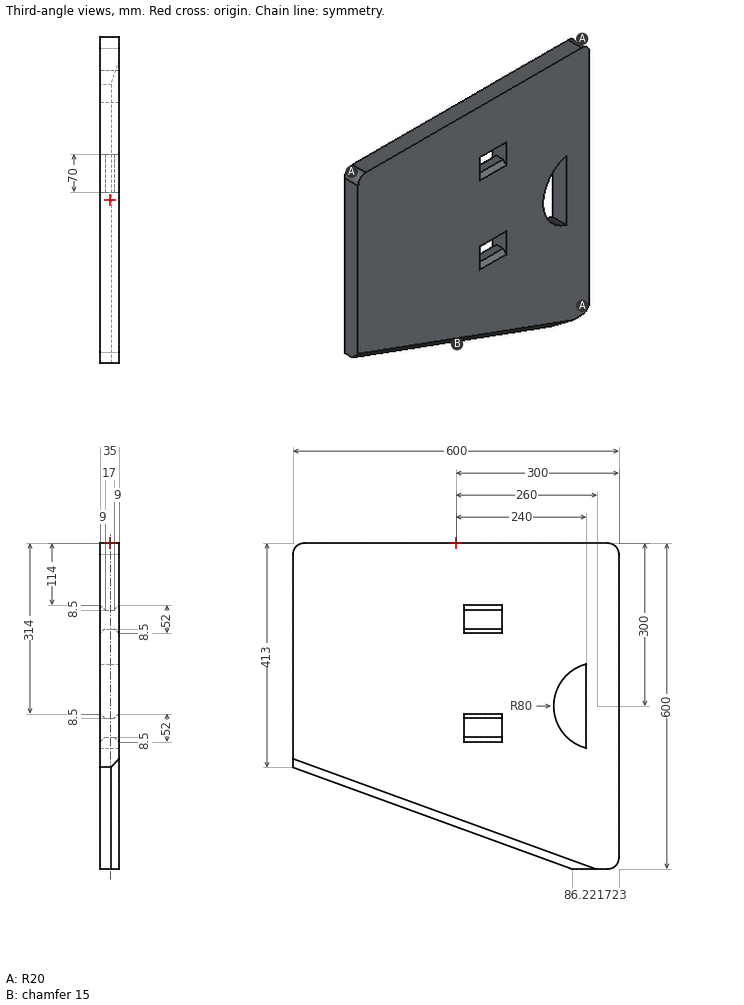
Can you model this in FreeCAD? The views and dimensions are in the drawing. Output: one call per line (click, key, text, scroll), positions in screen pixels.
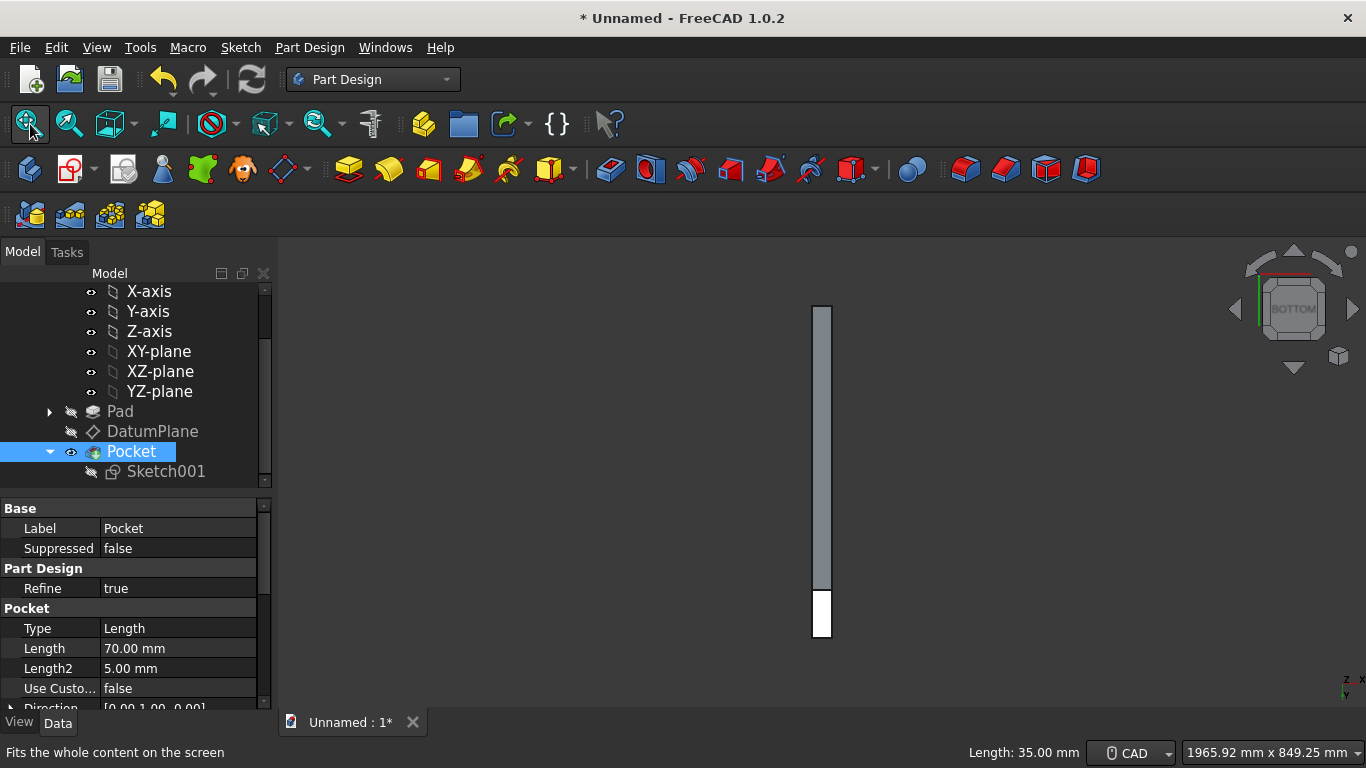
click(822, 637, ctrl)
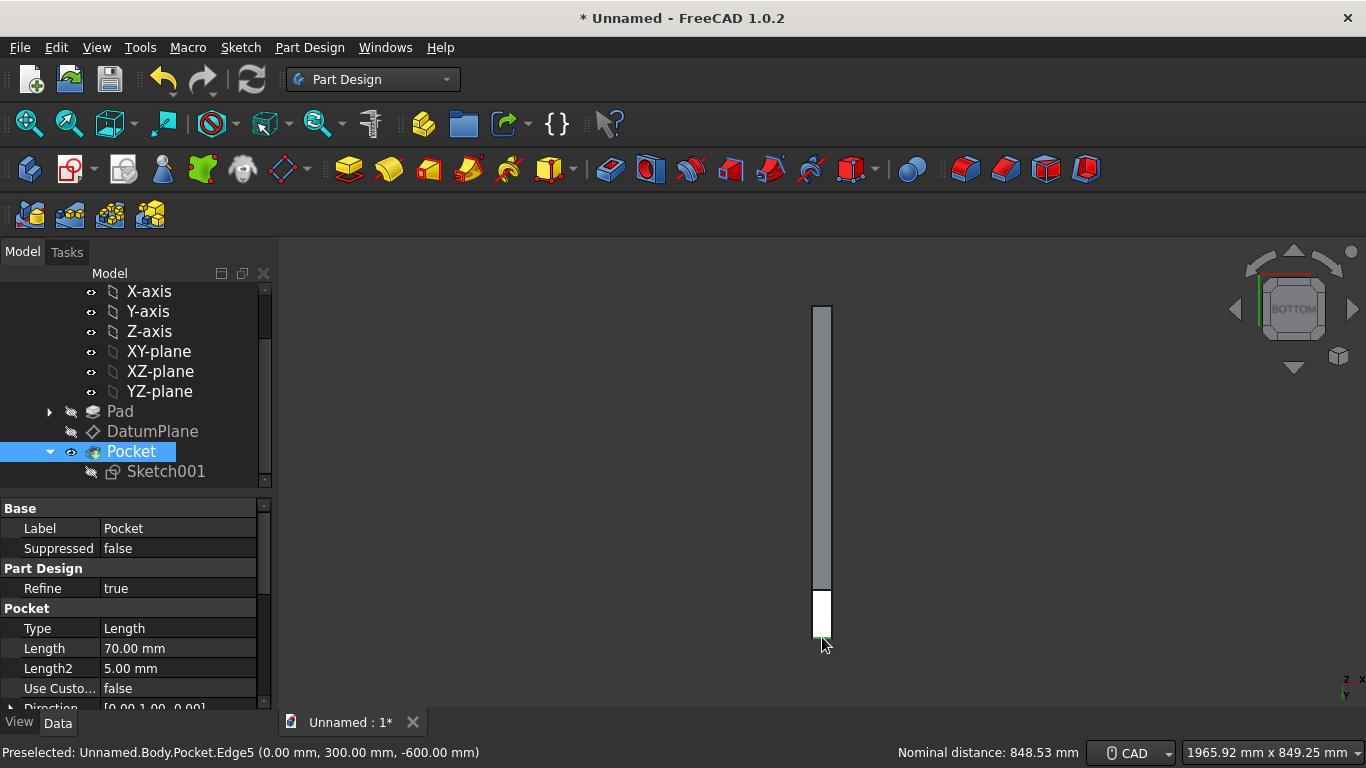
scroll(822, 637, up, 4)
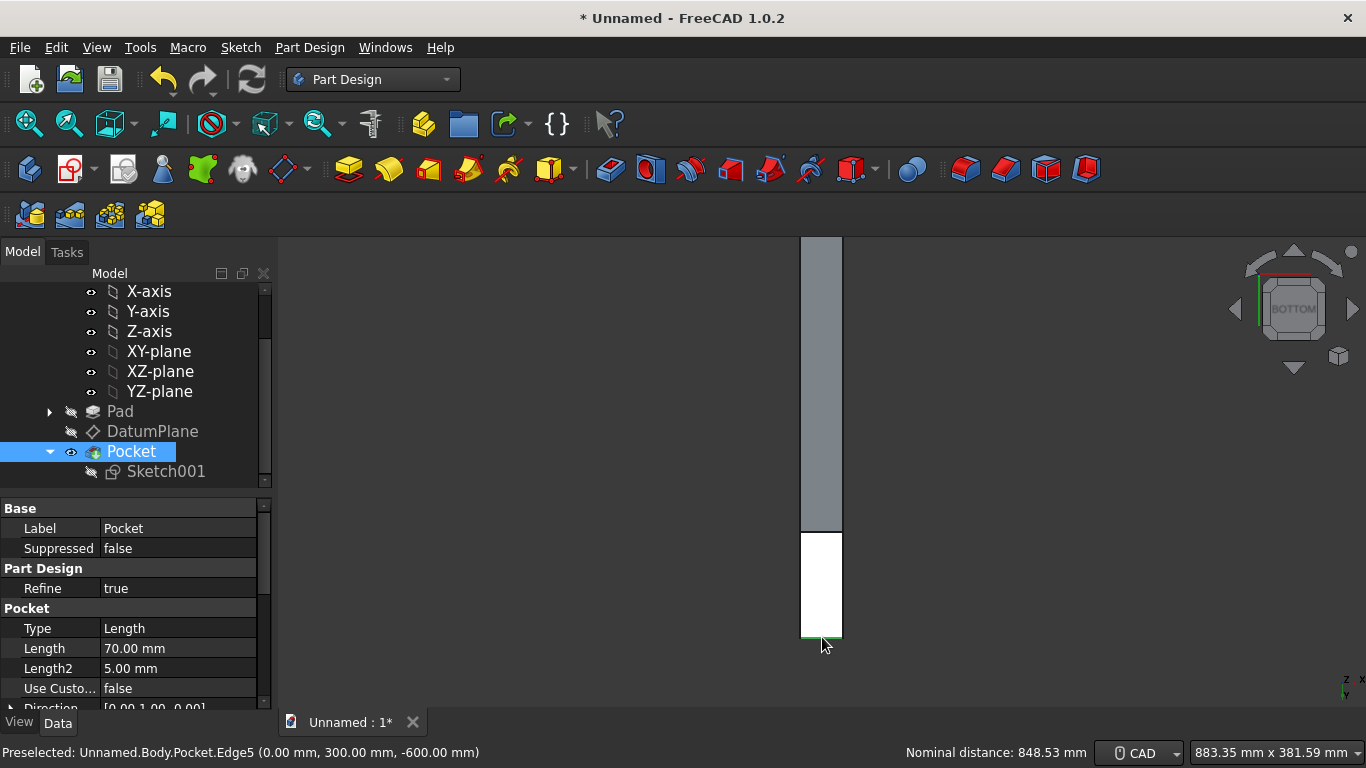
click(30, 124)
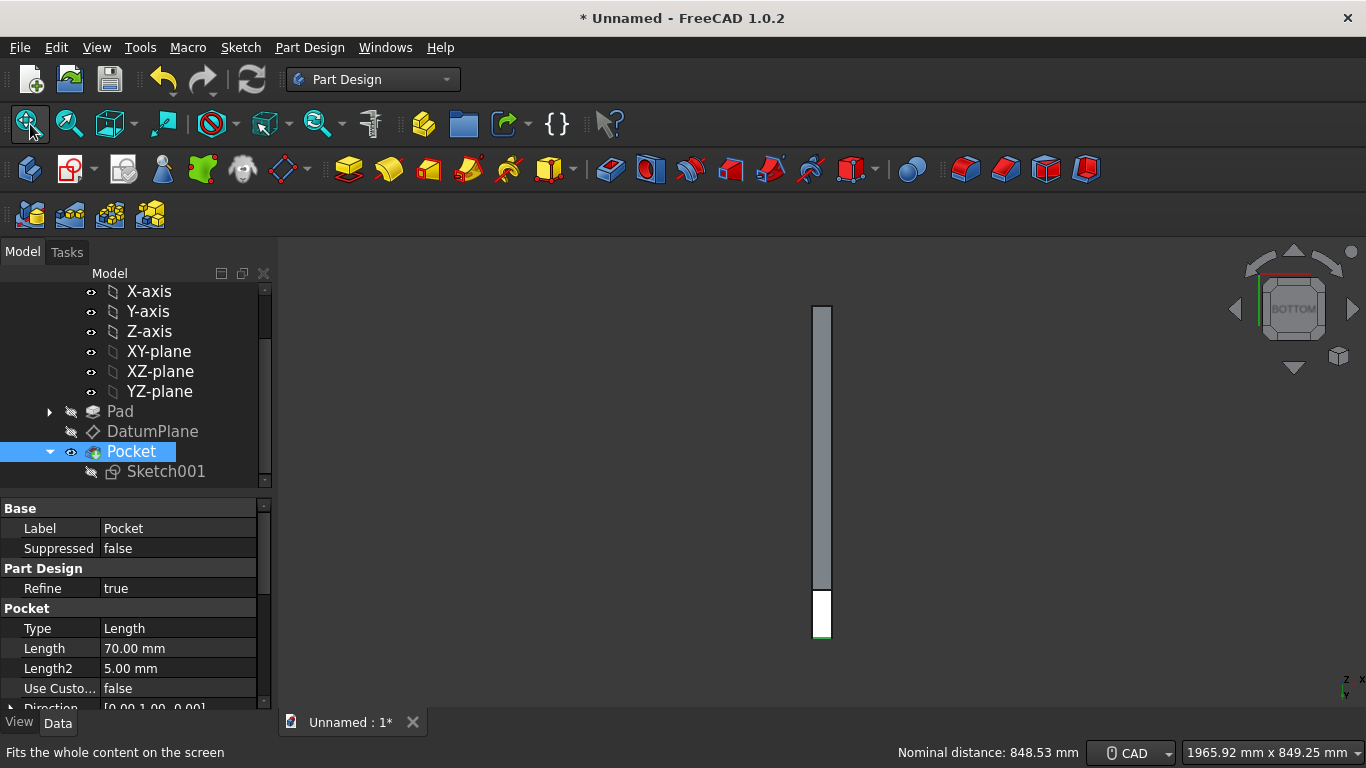
key(4)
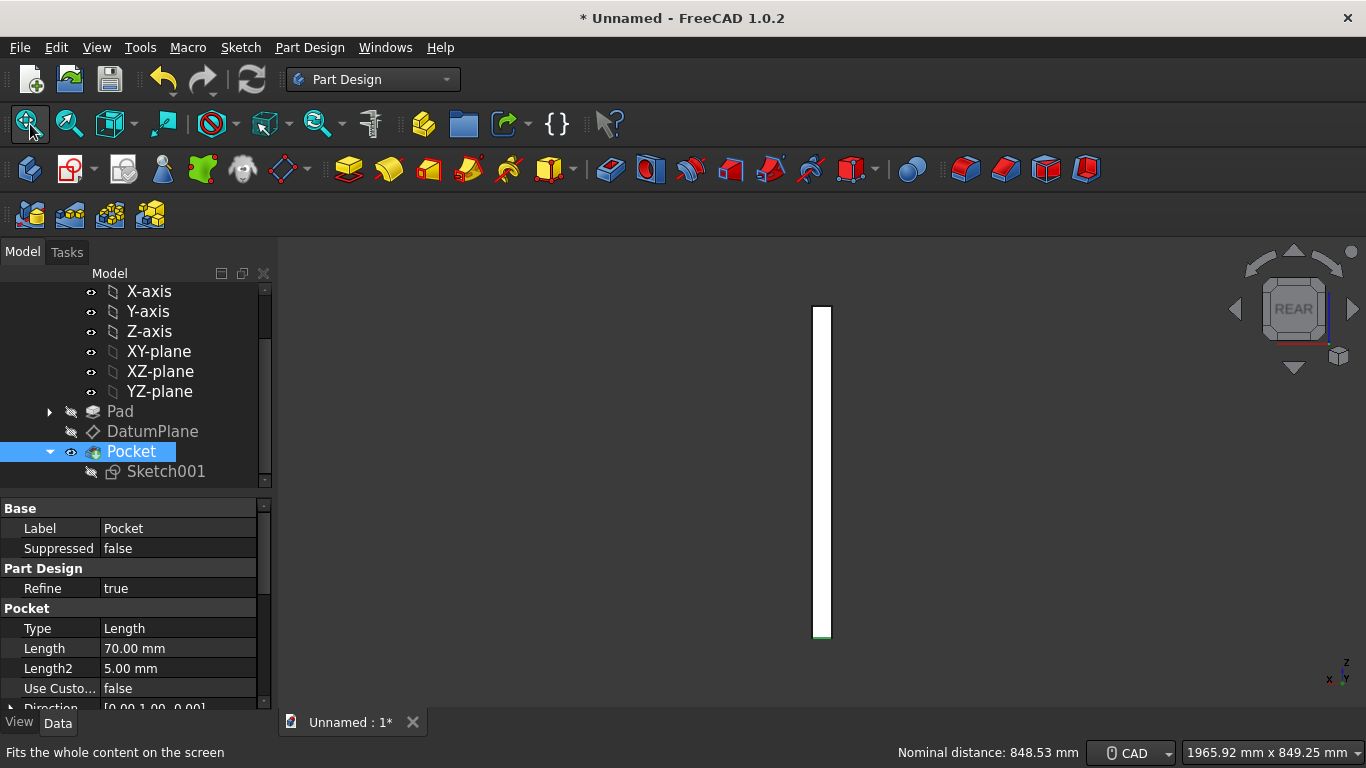
click(822, 305, ctrl)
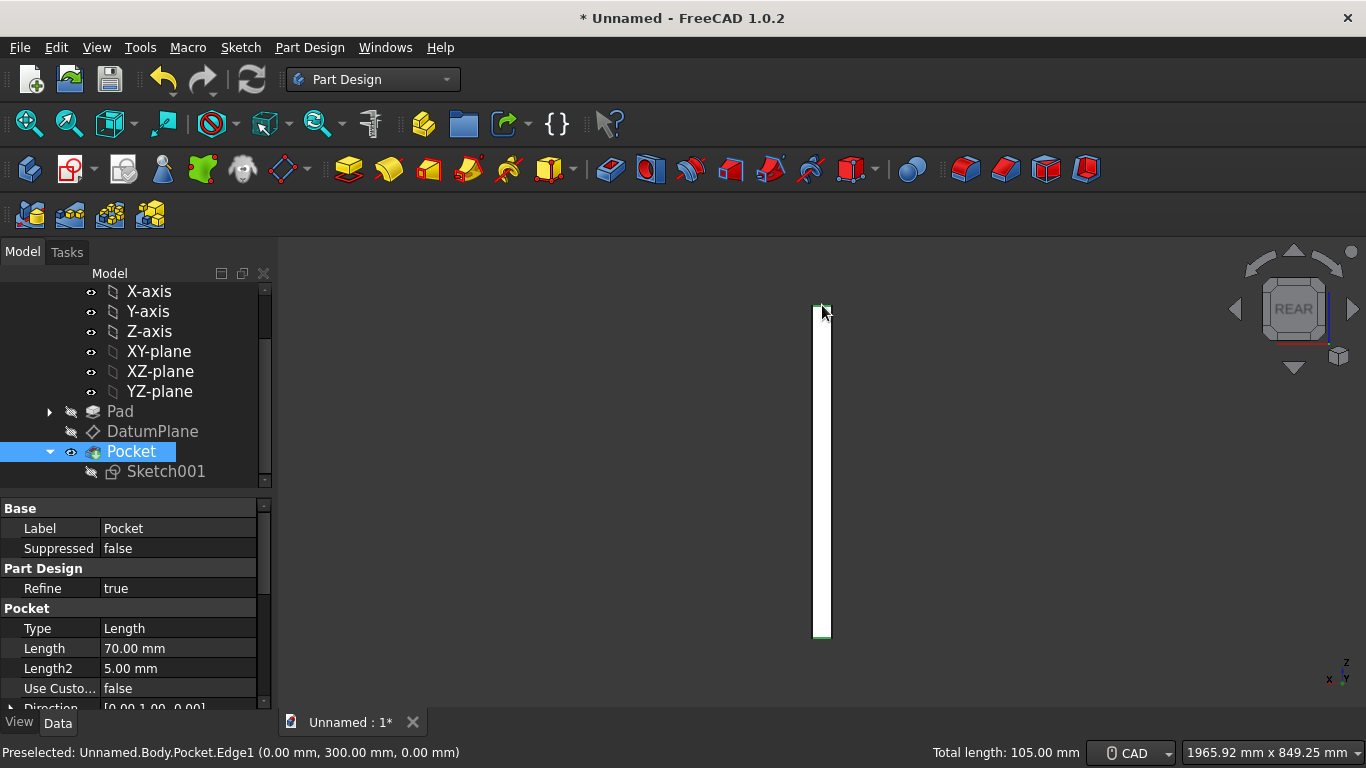
click(966, 170)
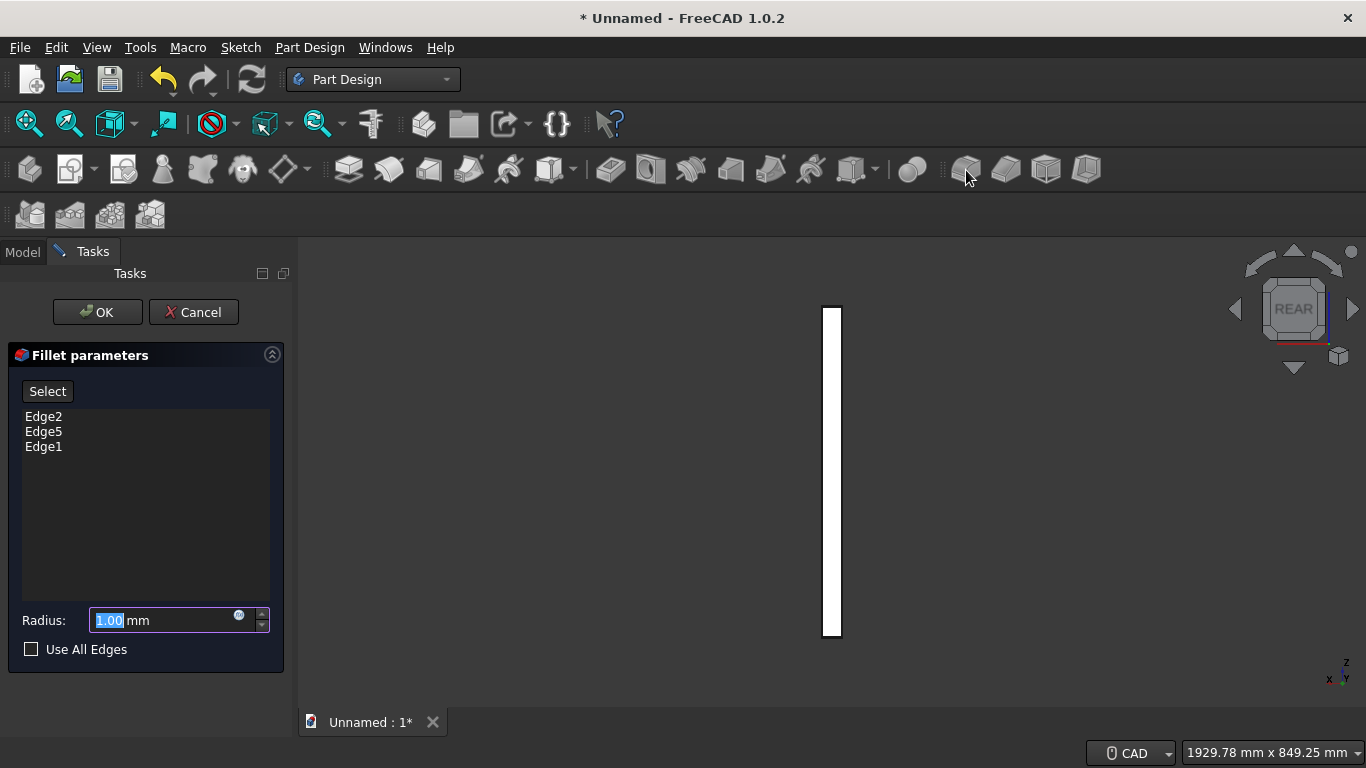
text(20)
key(Tab)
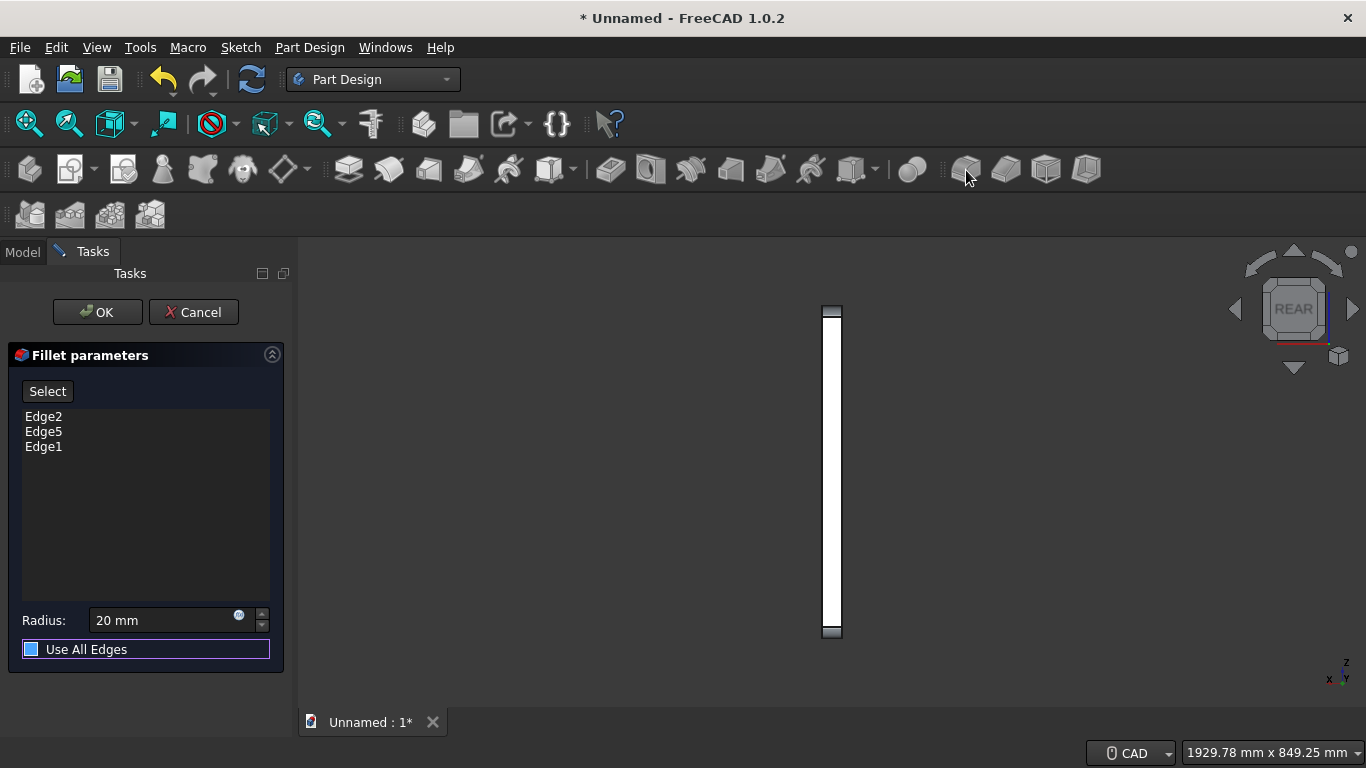
click(98, 312)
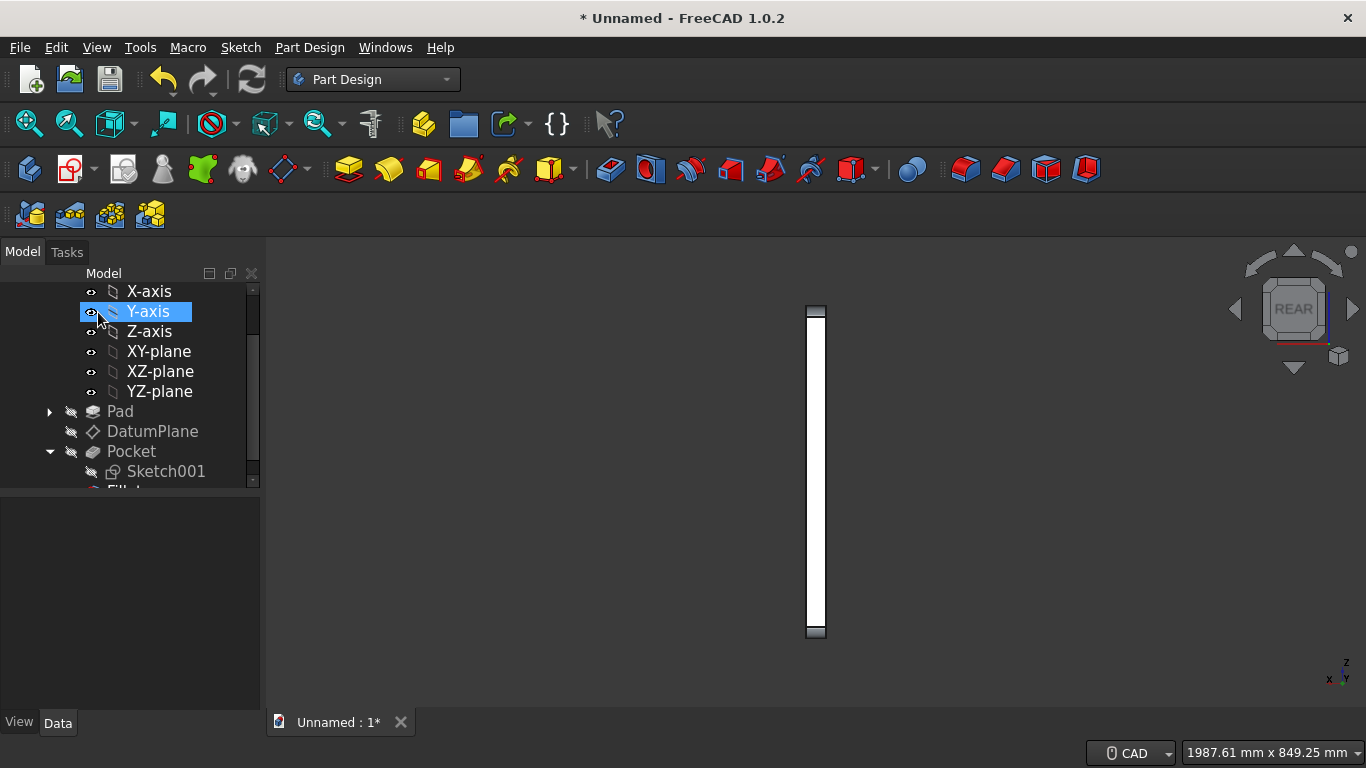
key(0)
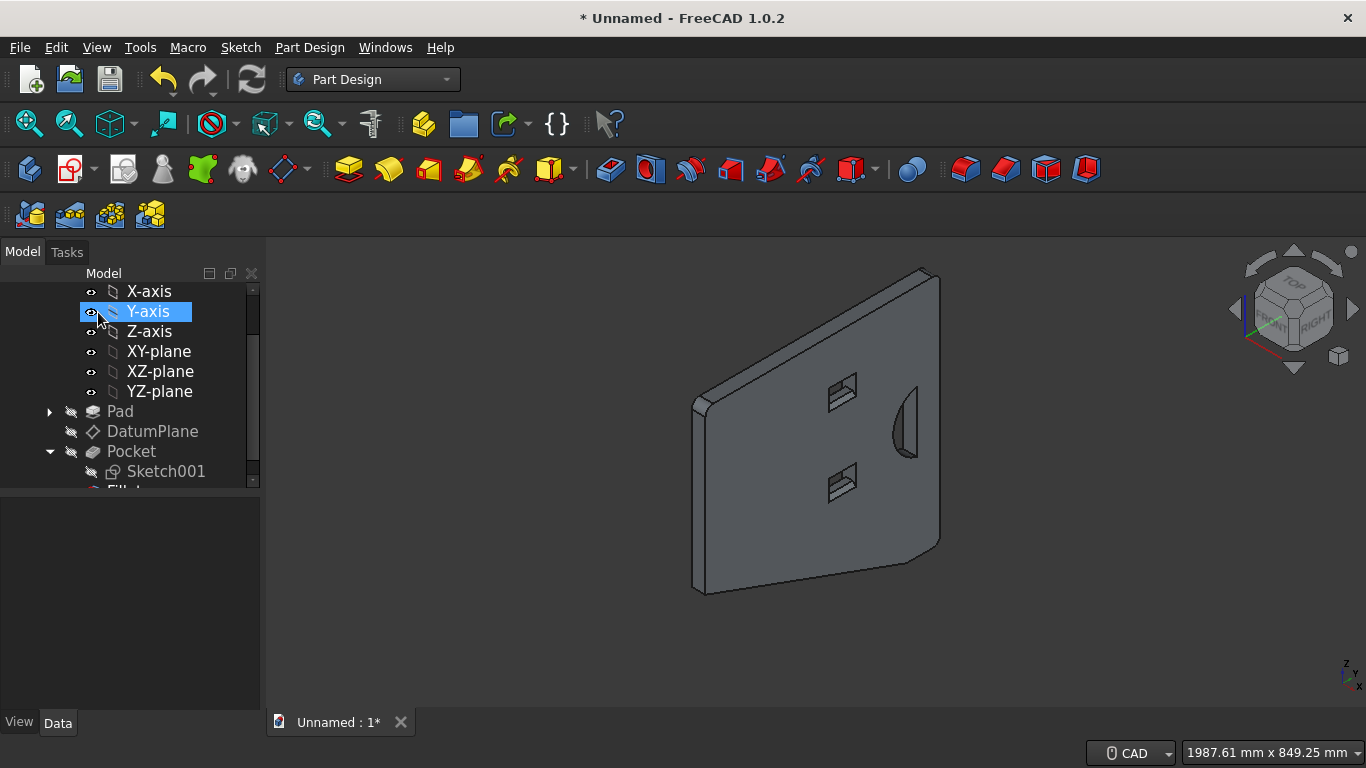
key(2)